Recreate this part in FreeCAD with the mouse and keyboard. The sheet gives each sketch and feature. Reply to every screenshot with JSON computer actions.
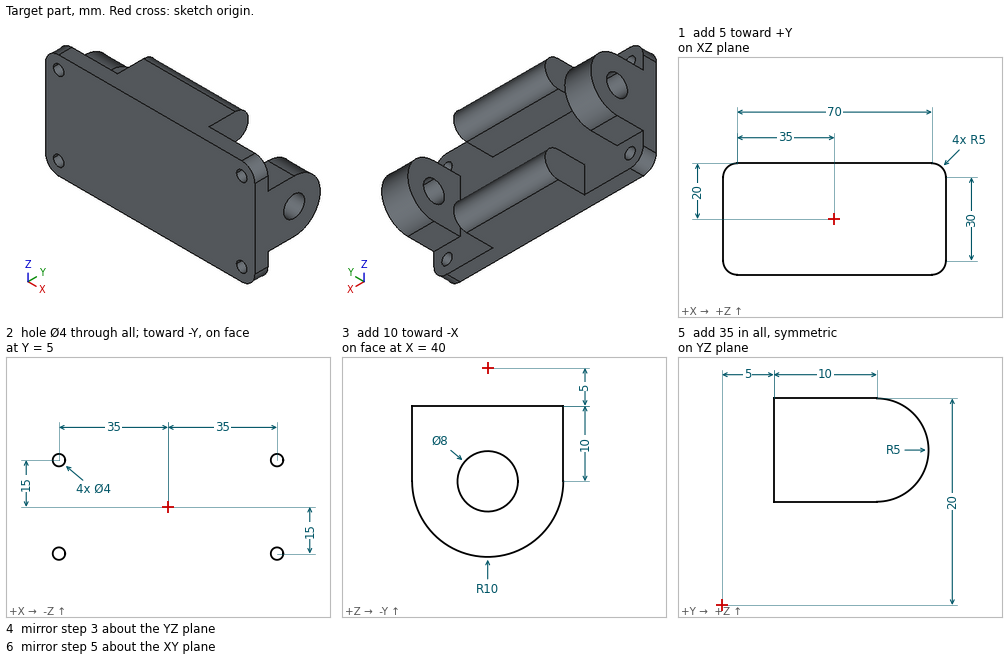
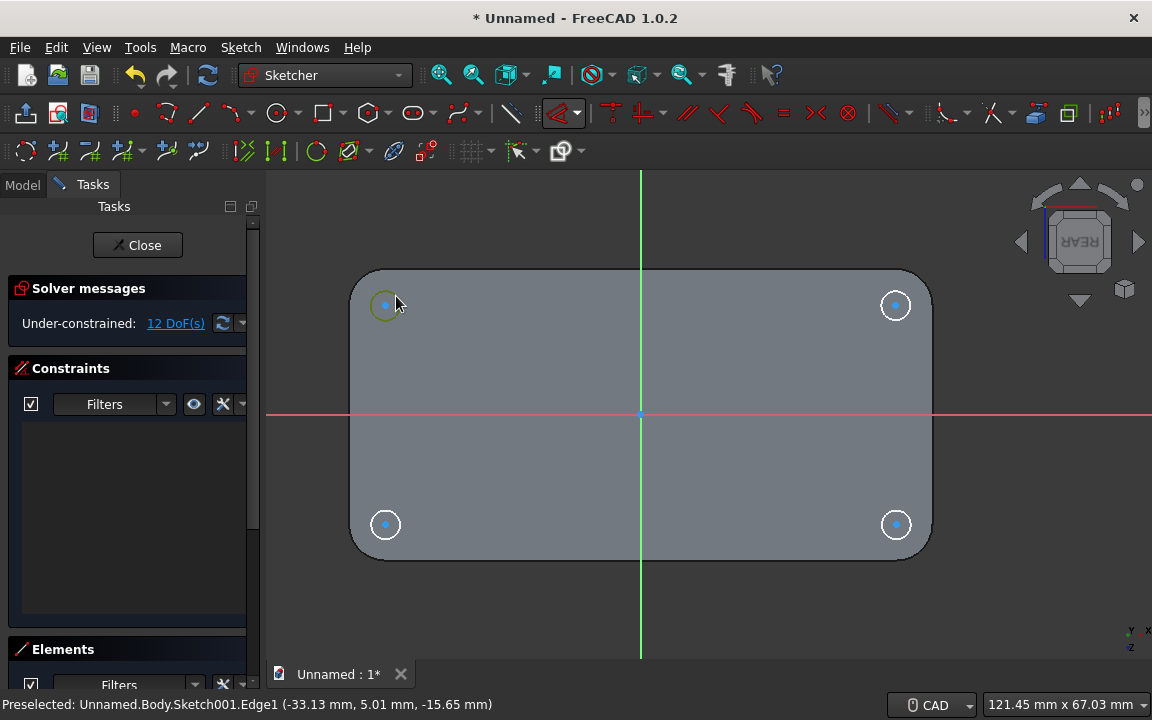
{"action": "left_click", "coordinate": [906, 295]}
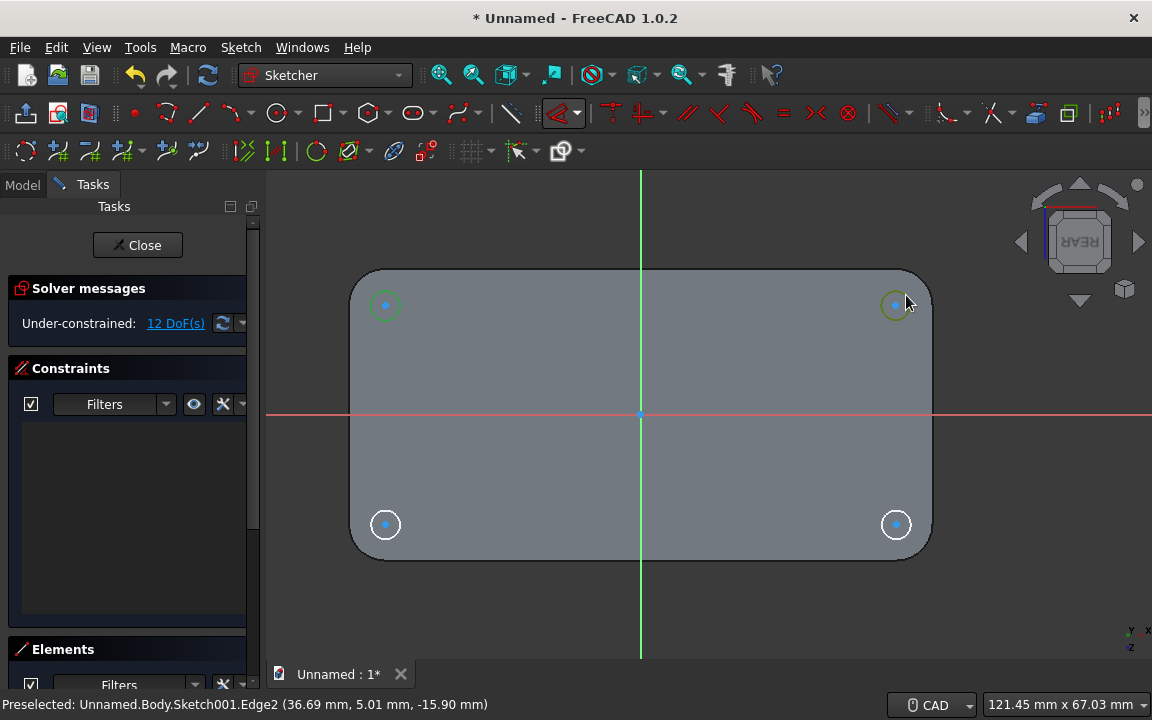
{"action": "left_click", "coordinate": [906, 515]}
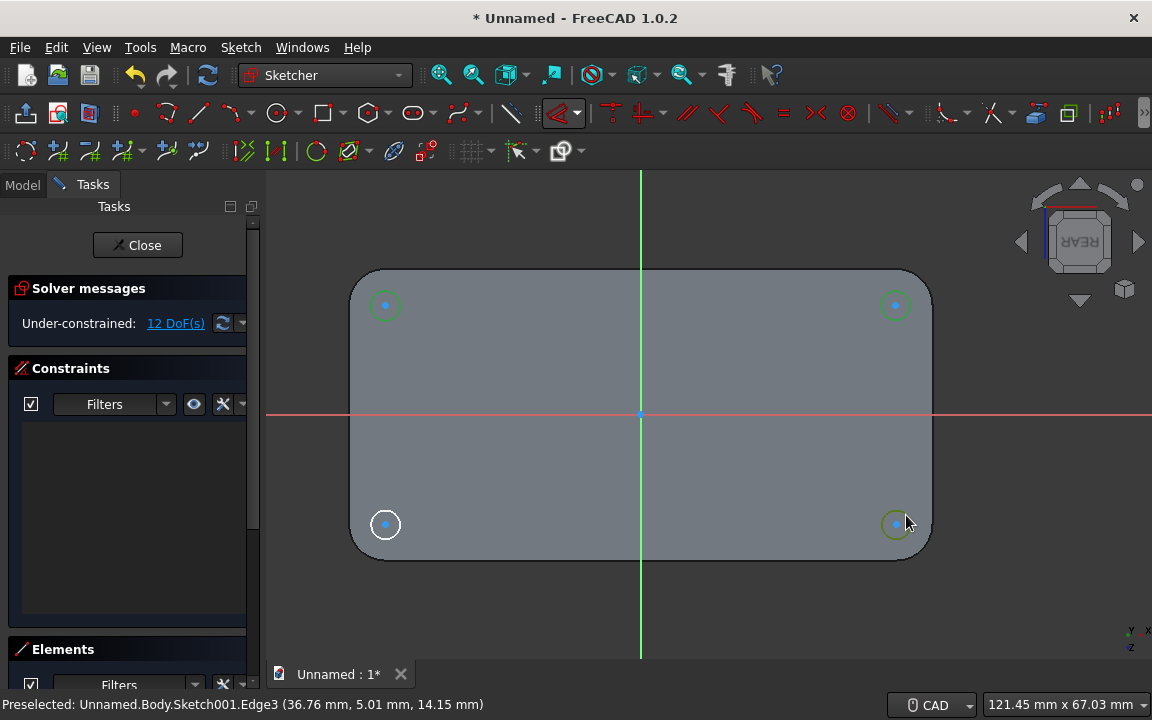
{"action": "left_click", "coordinate": [396, 515]}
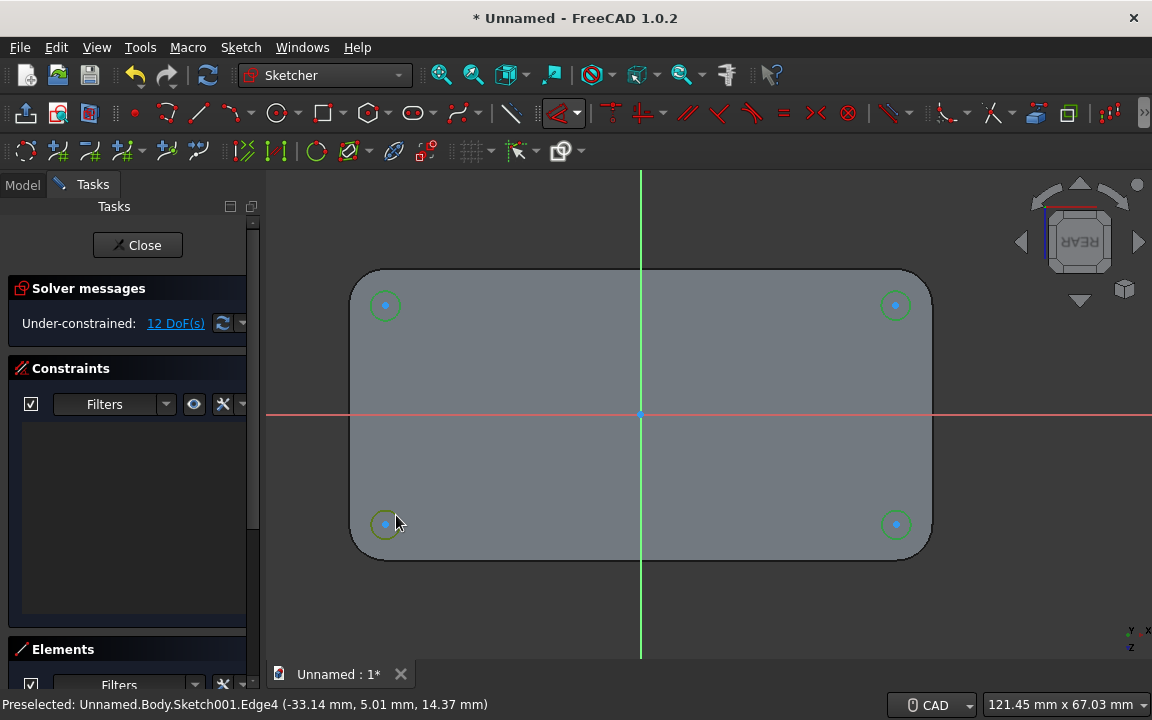
{"action": "key", "text": "e"}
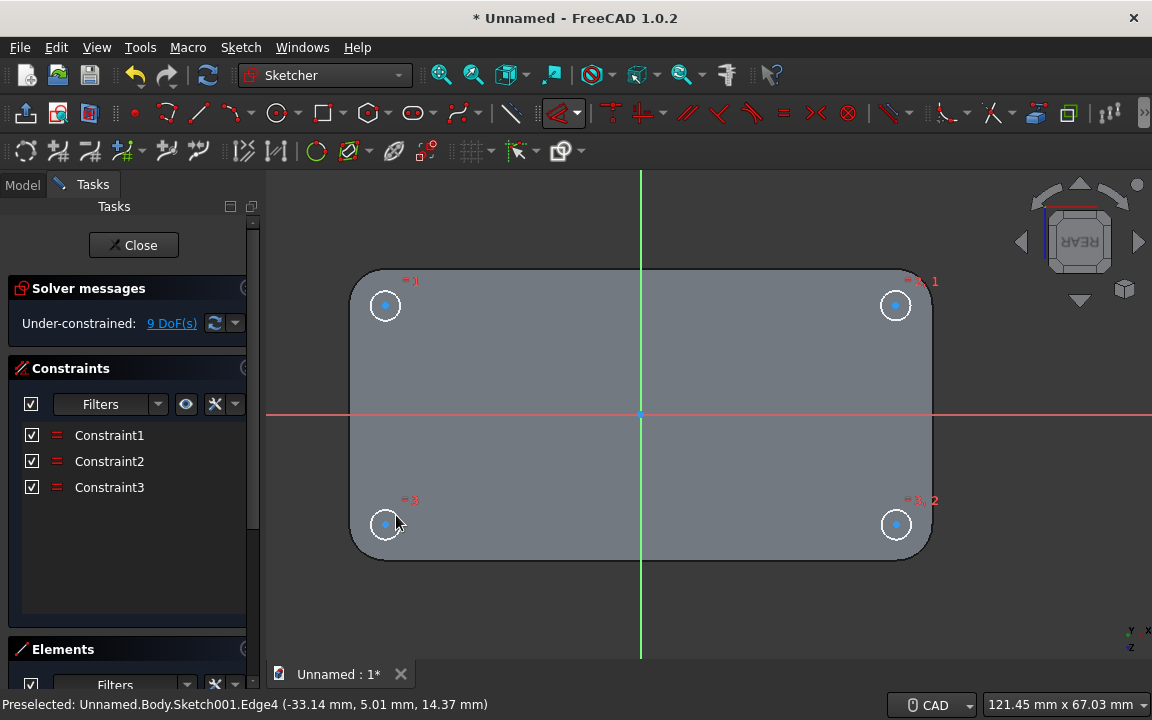
{"action": "left_click", "coordinate": [385, 306]}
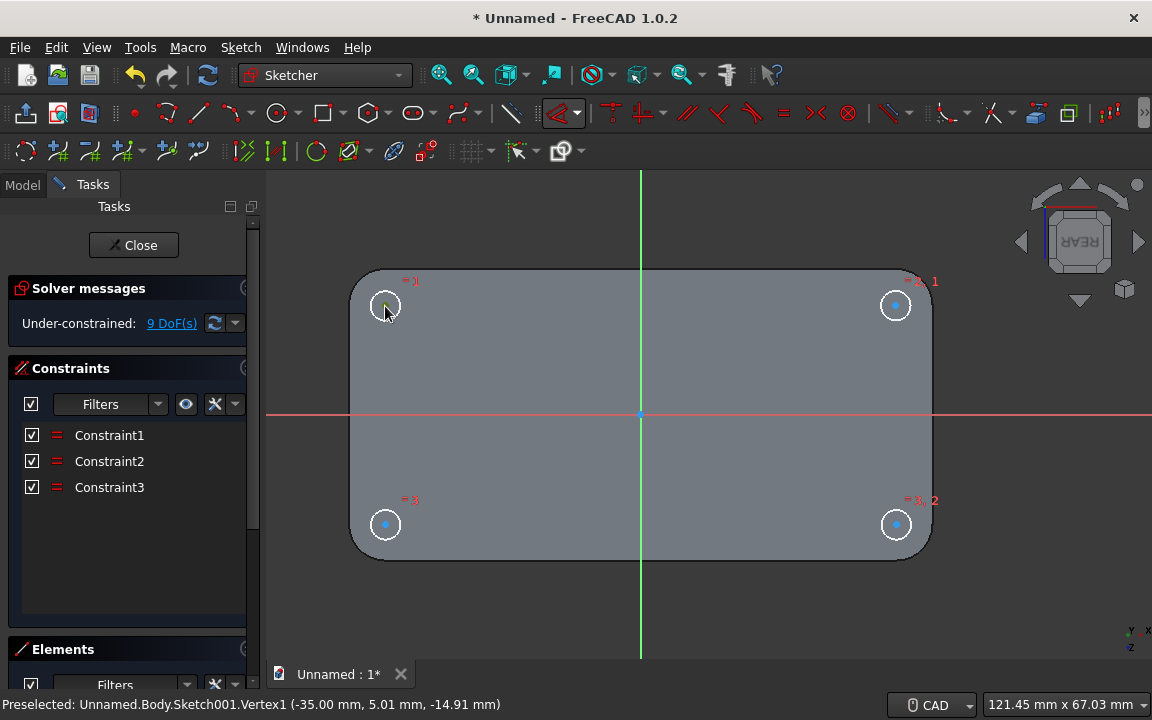
{"action": "left_click", "coordinate": [896, 306]}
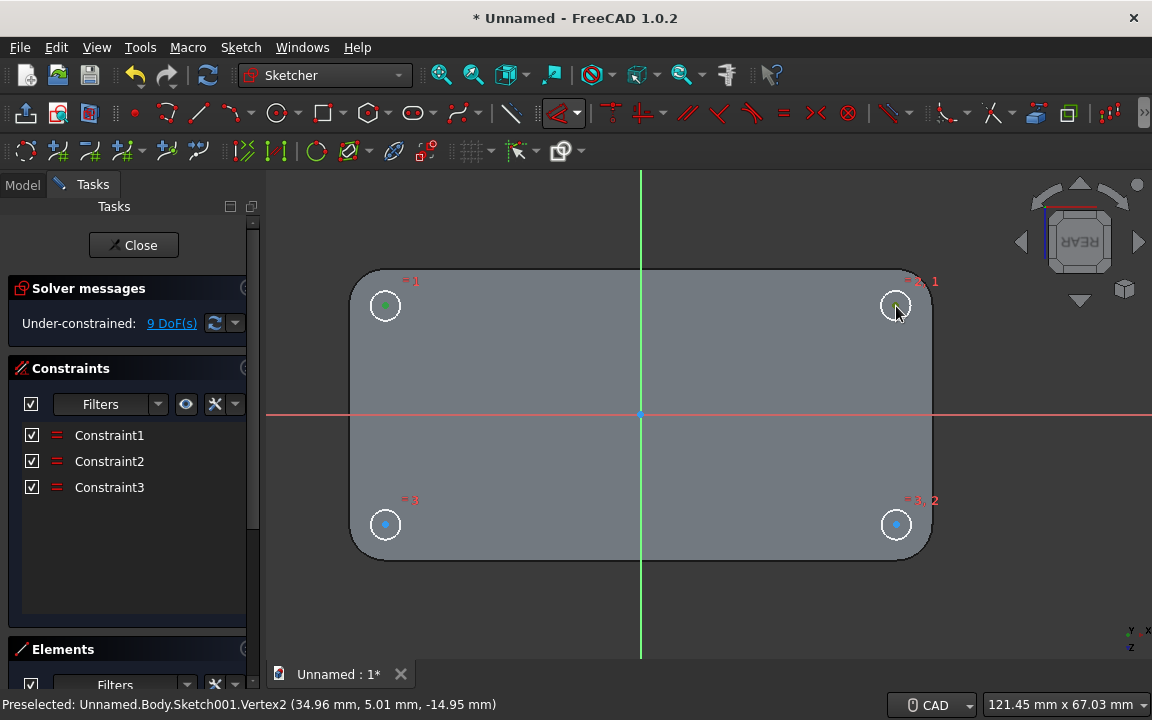
{"action": "left_click", "coordinate": [666, 114]}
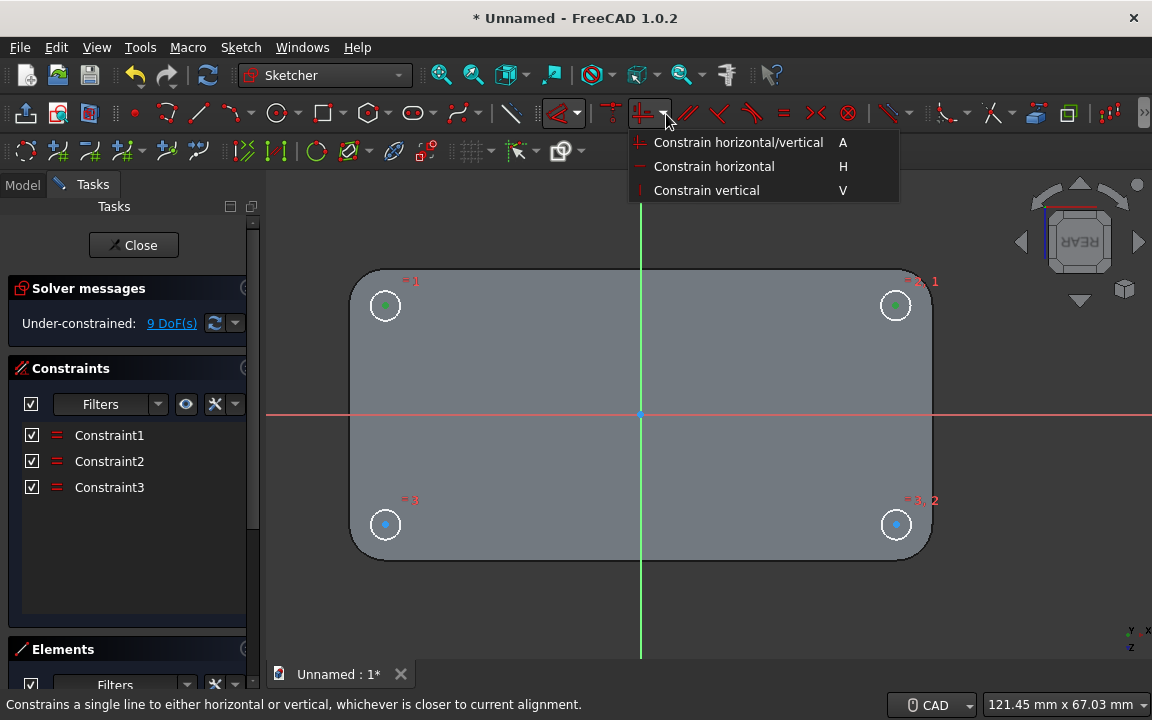
{"action": "left_click", "coordinate": [764, 166]}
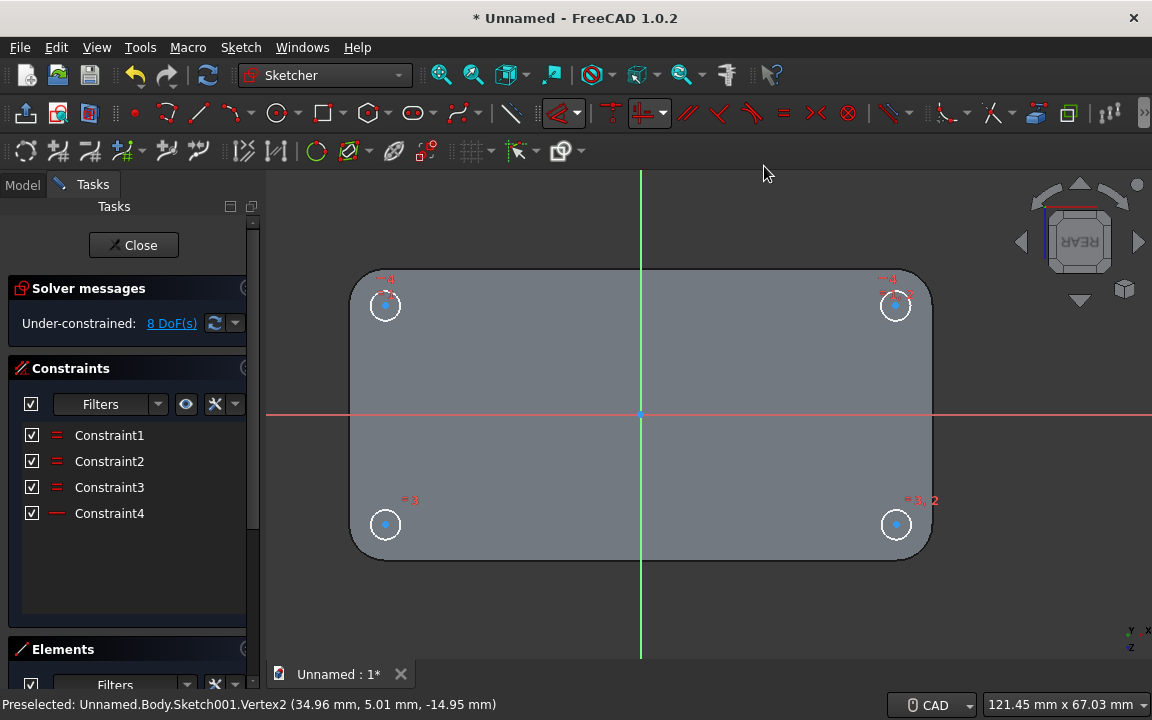
{"action": "left_click", "coordinate": [896, 306]}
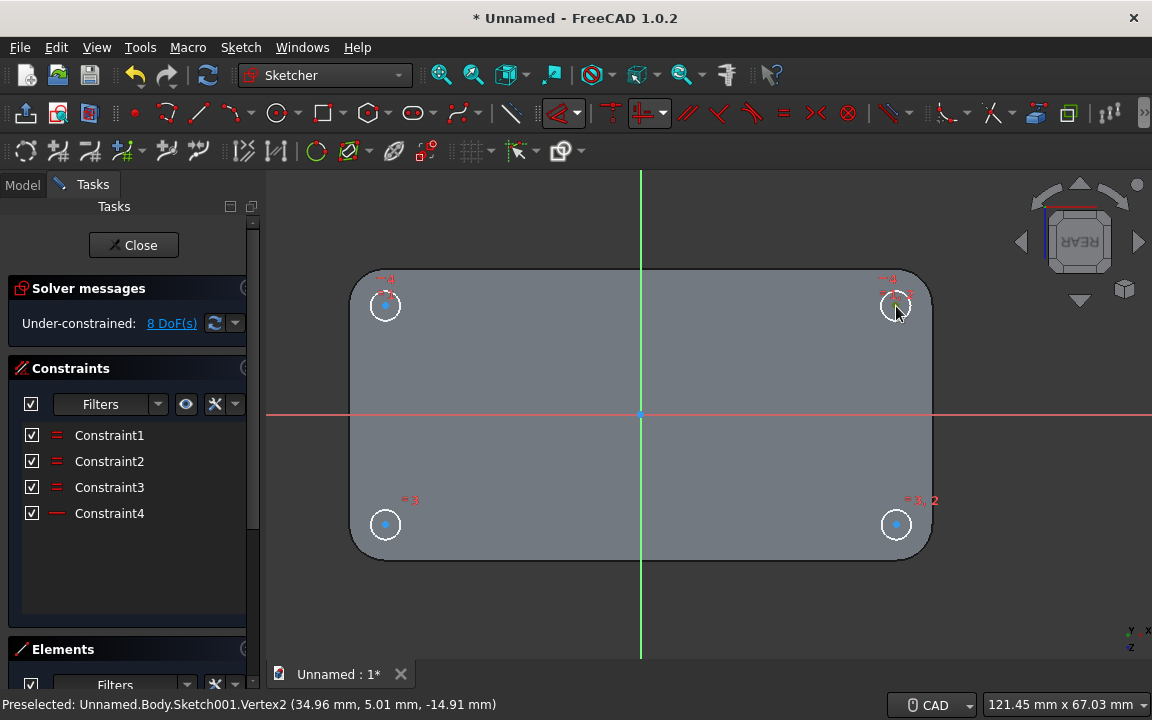
{"action": "left_click", "coordinate": [896, 525]}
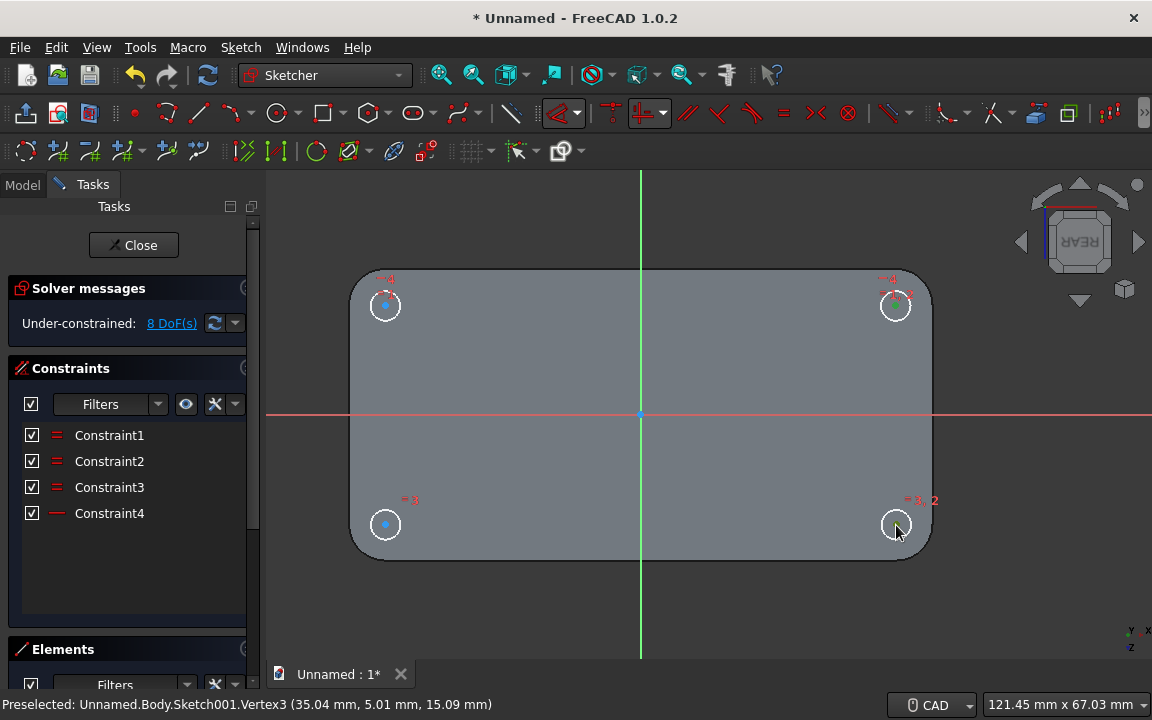
{"action": "key", "text": "v"}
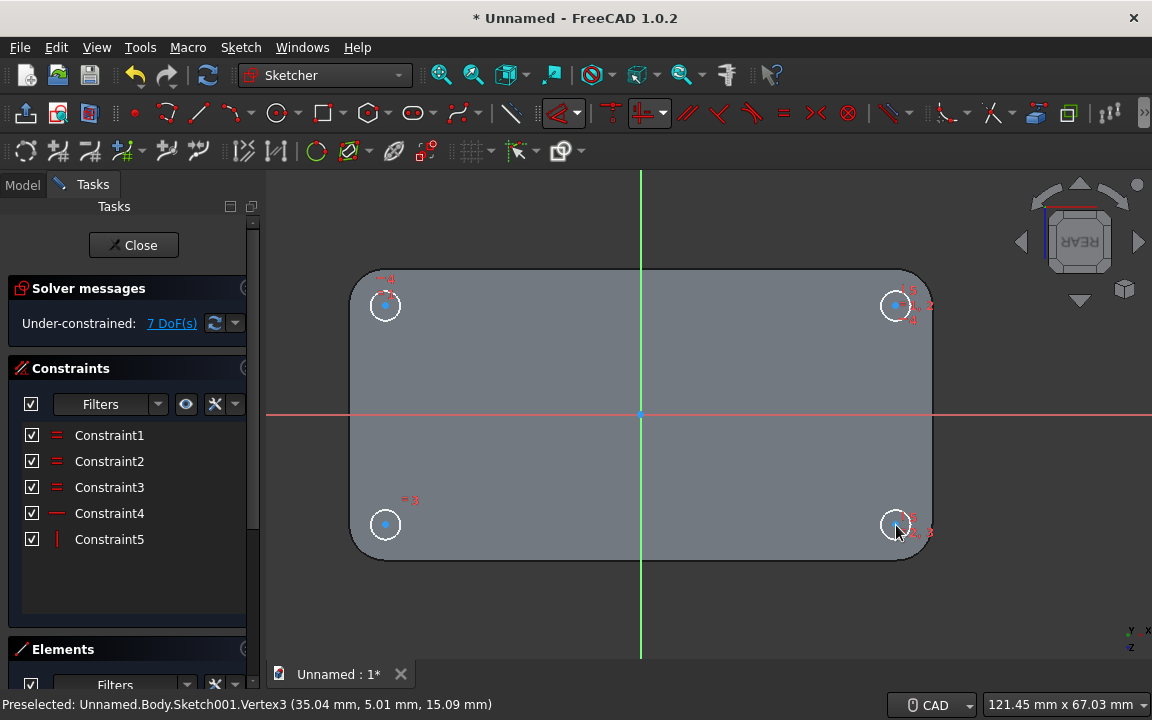
{"action": "left_click", "coordinate": [385, 306]}